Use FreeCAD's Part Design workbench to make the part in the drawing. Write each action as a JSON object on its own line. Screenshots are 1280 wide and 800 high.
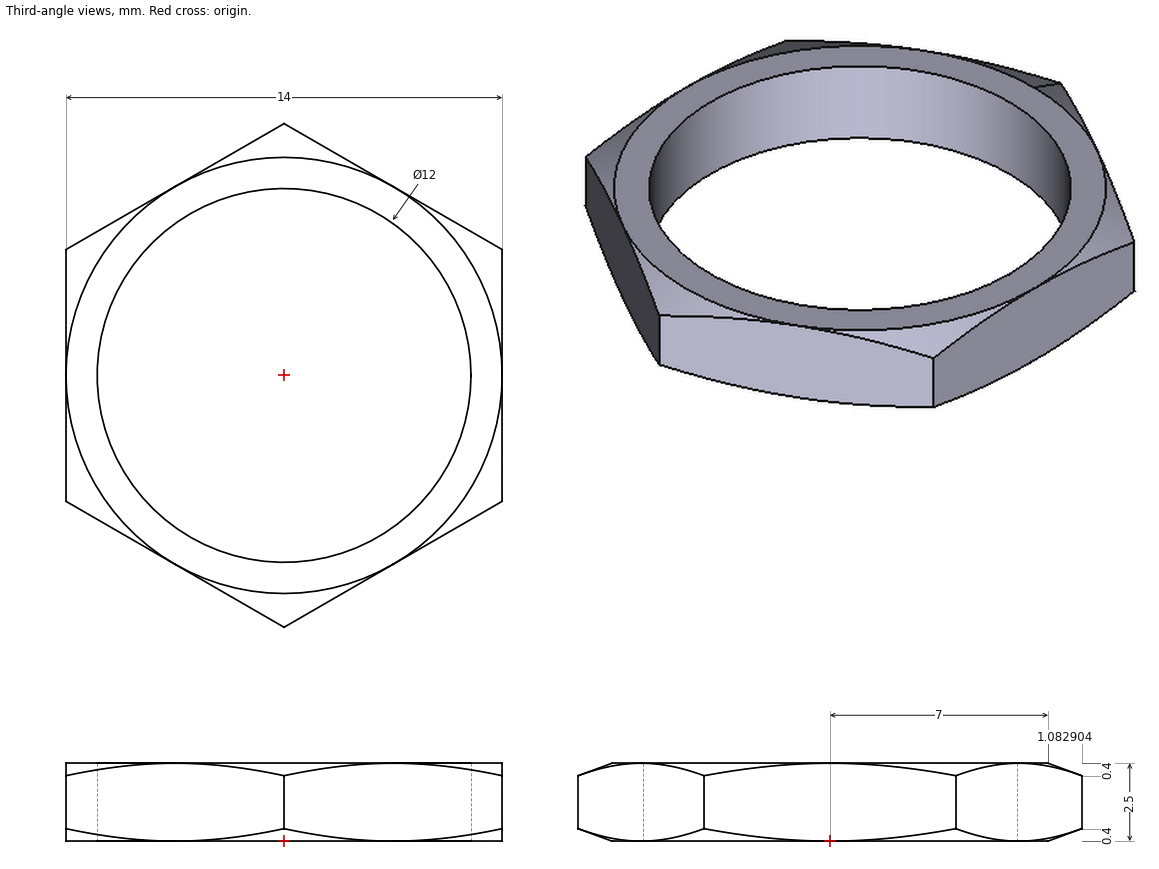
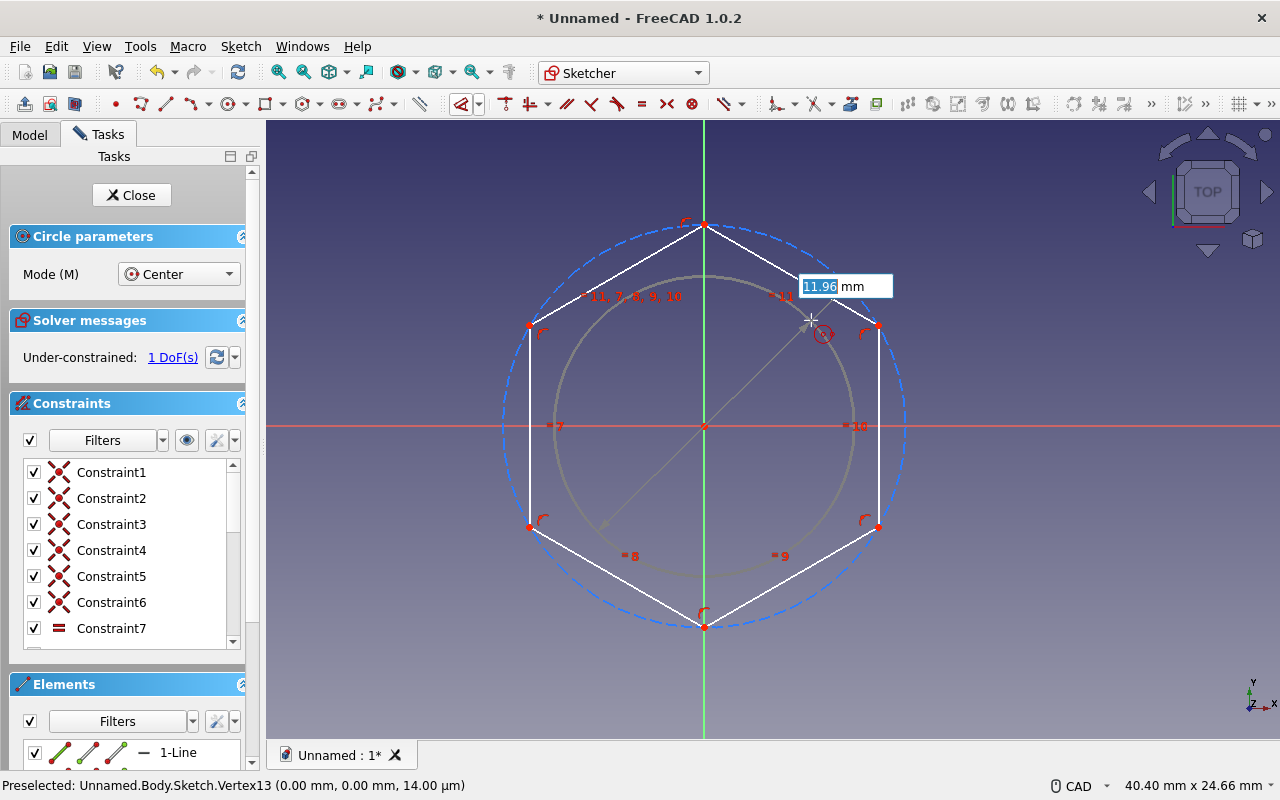
{"action": "type", "text": "12"}
{"action": "key", "text": "Return"}
{"action": "key", "text": "Escape"}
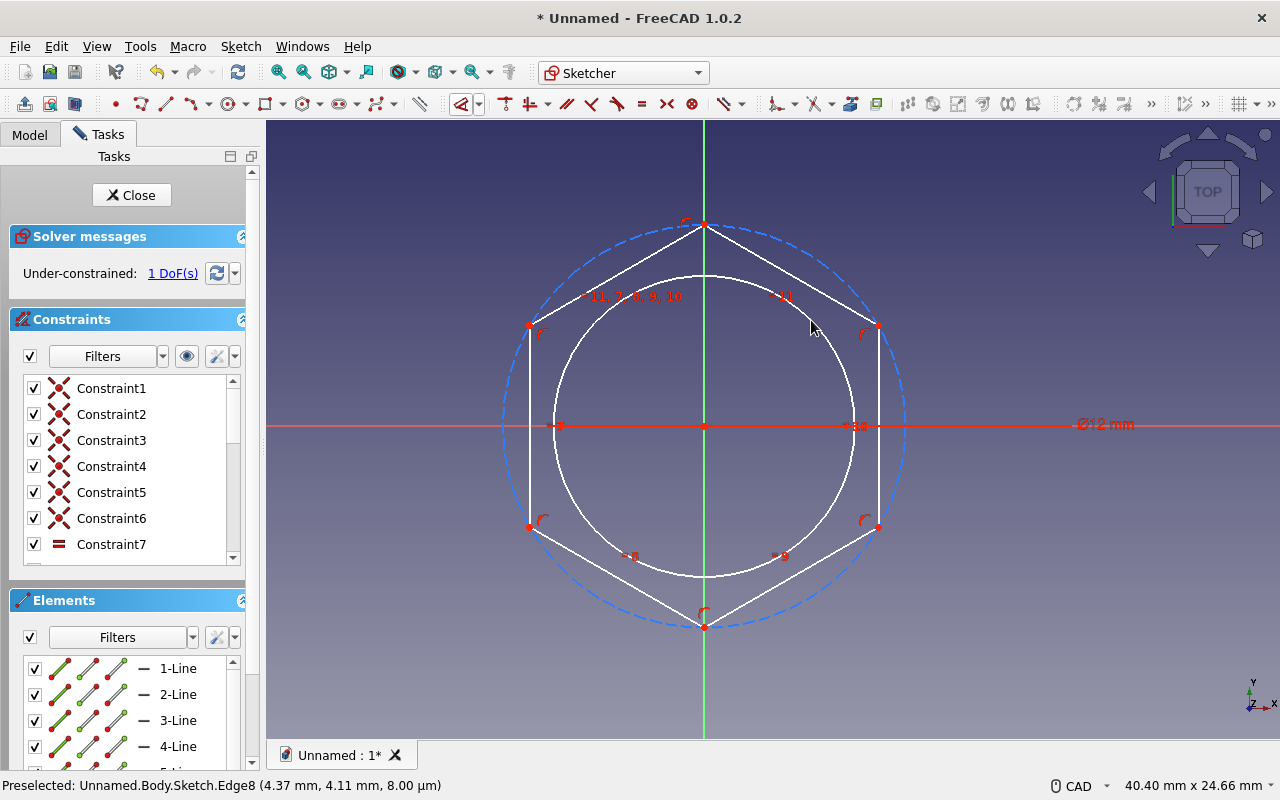
{"action": "left_click", "coordinate": [460, 104]}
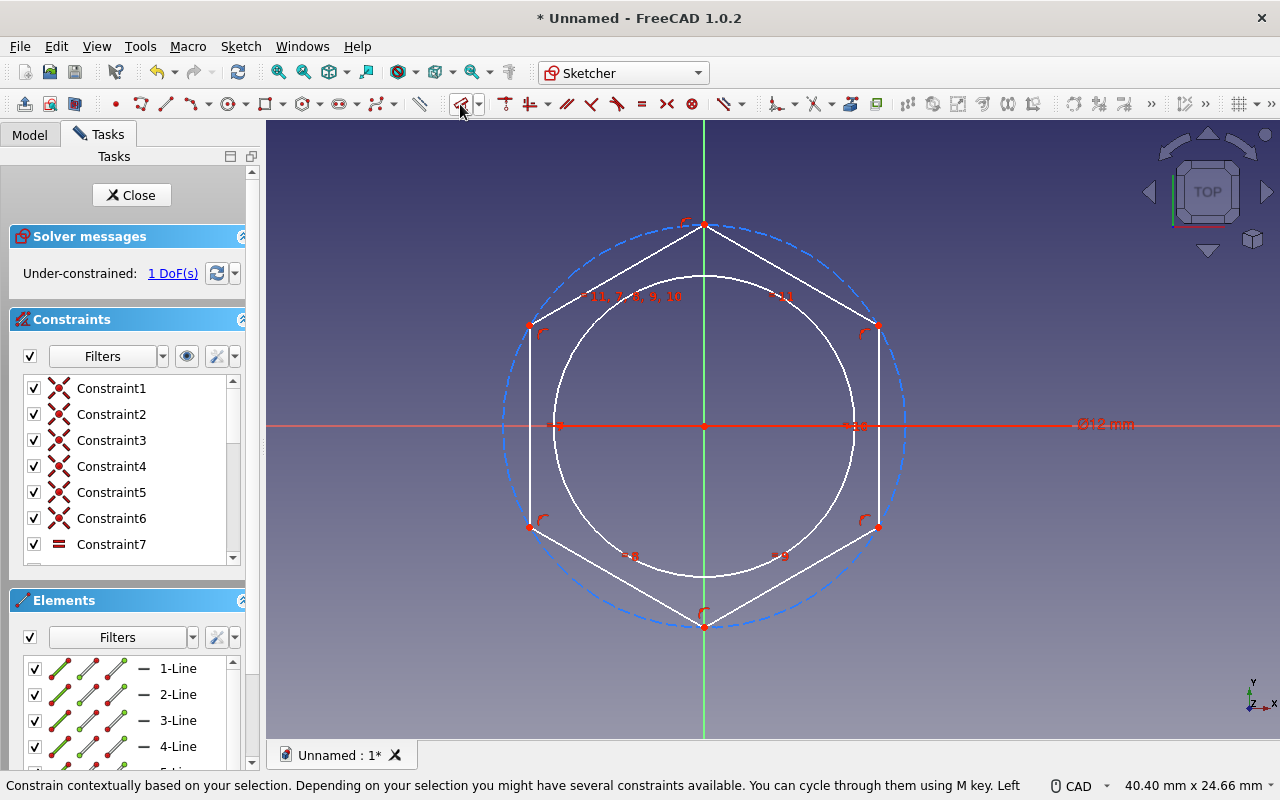
{"action": "left_click", "coordinate": [530, 326]}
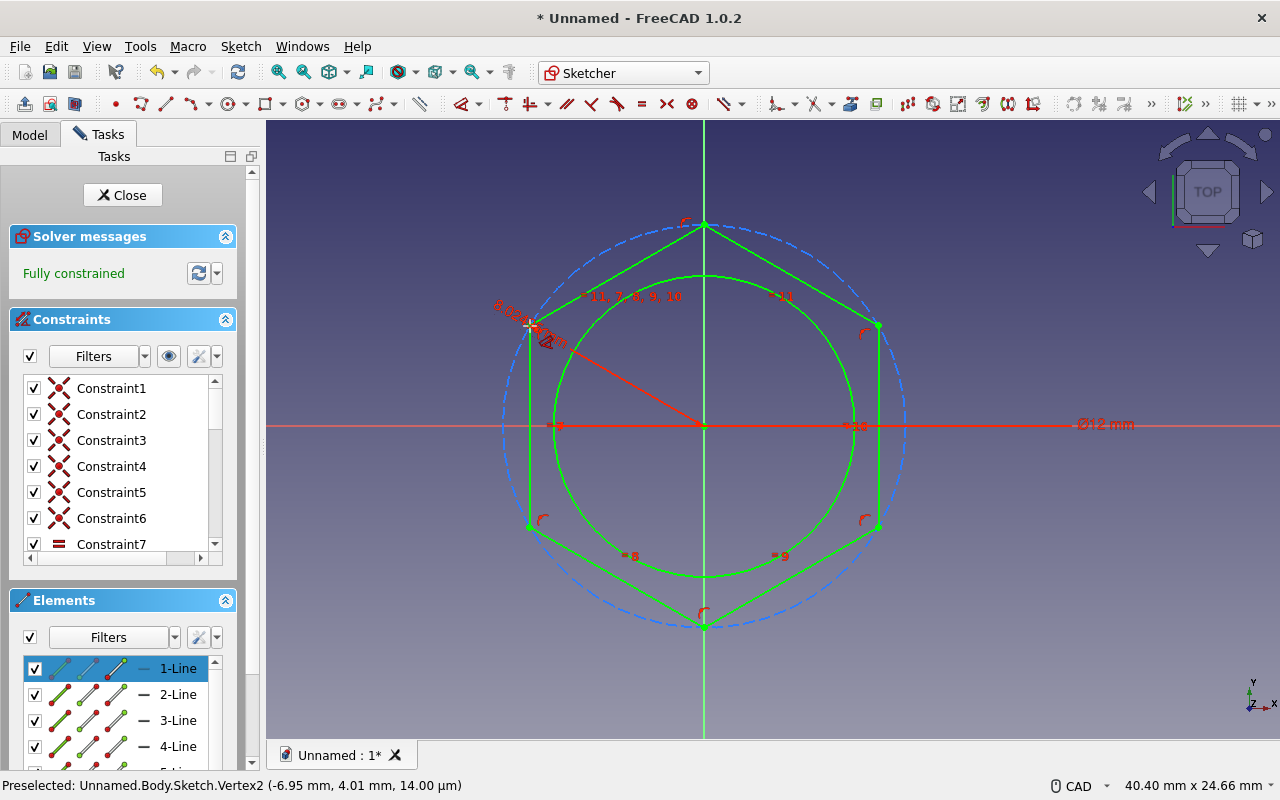
{"action": "left_click", "coordinate": [879, 527]}
{"action": "left_click", "coordinate": [582, 609]}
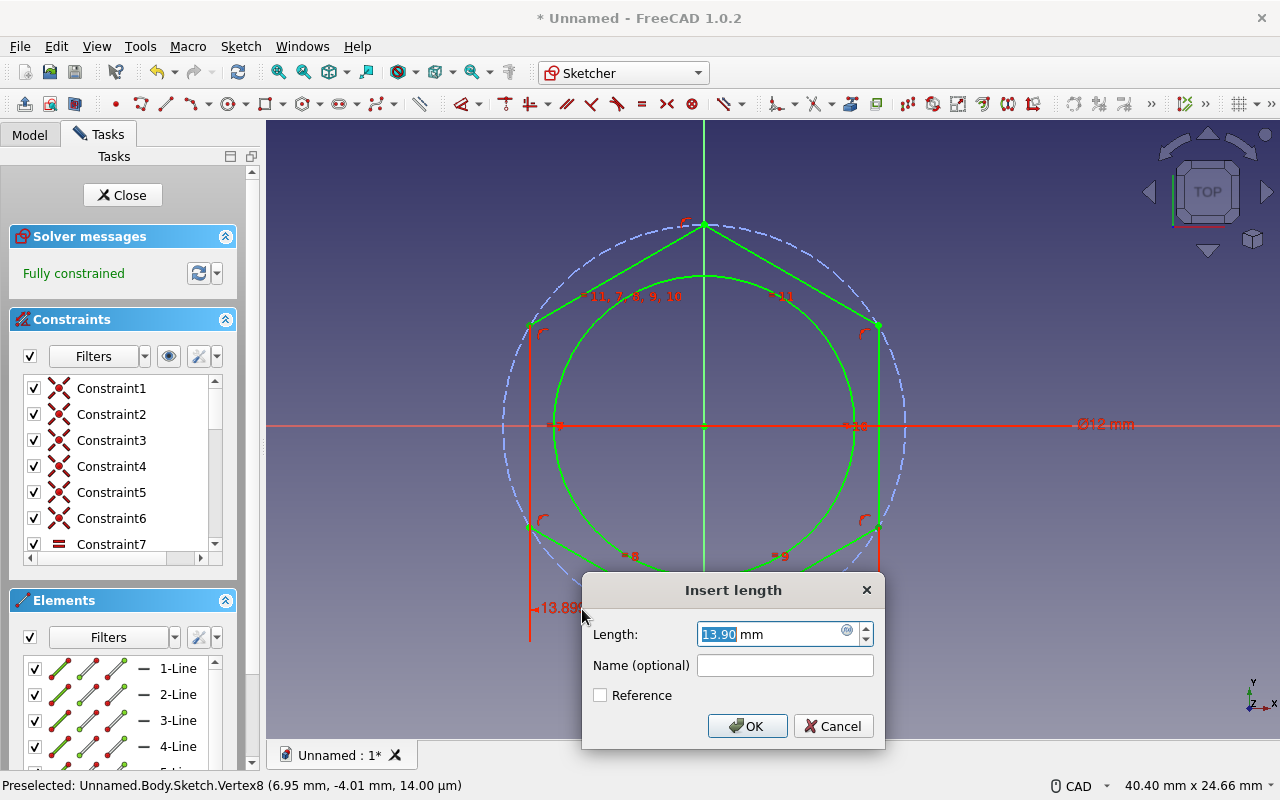
{"action": "type", "text": "14"}
{"action": "key", "text": "Return"}
{"action": "key", "text": "Escape"}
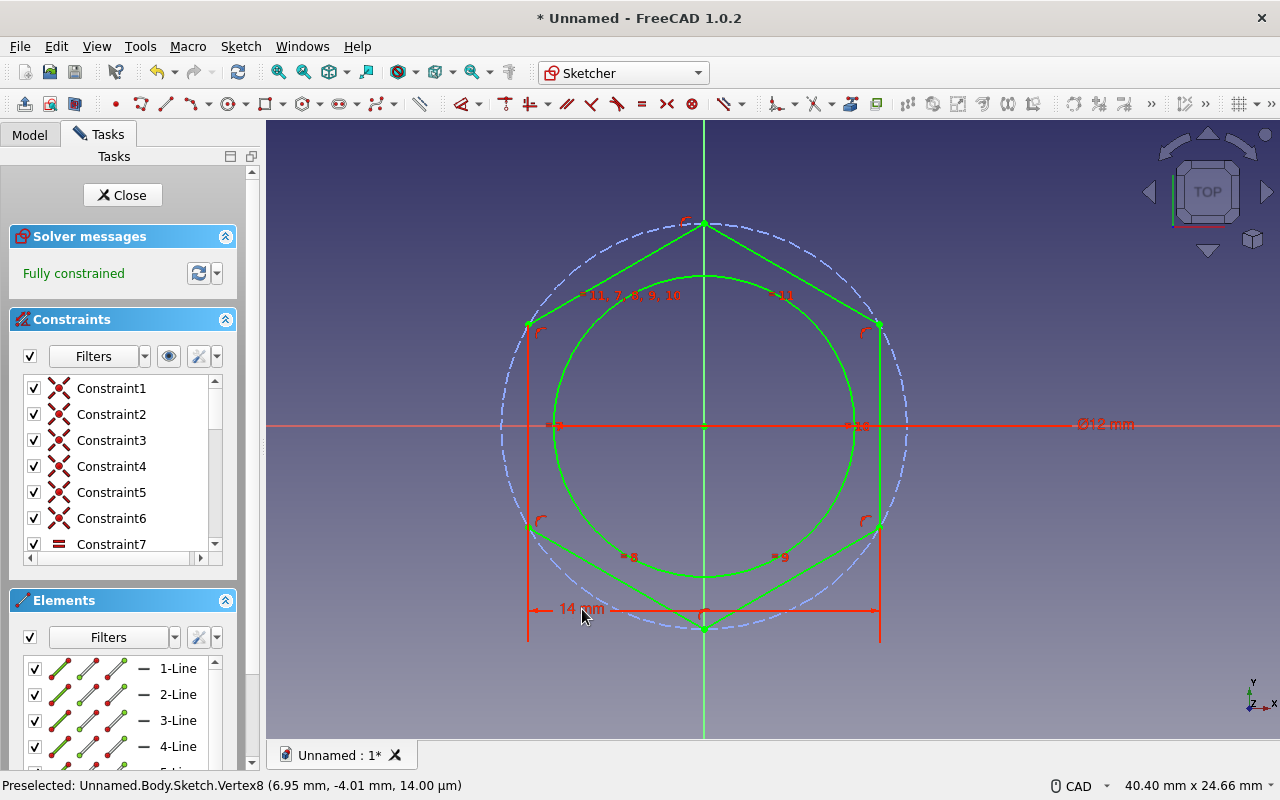
{"action": "left_click", "coordinate": [123, 195]}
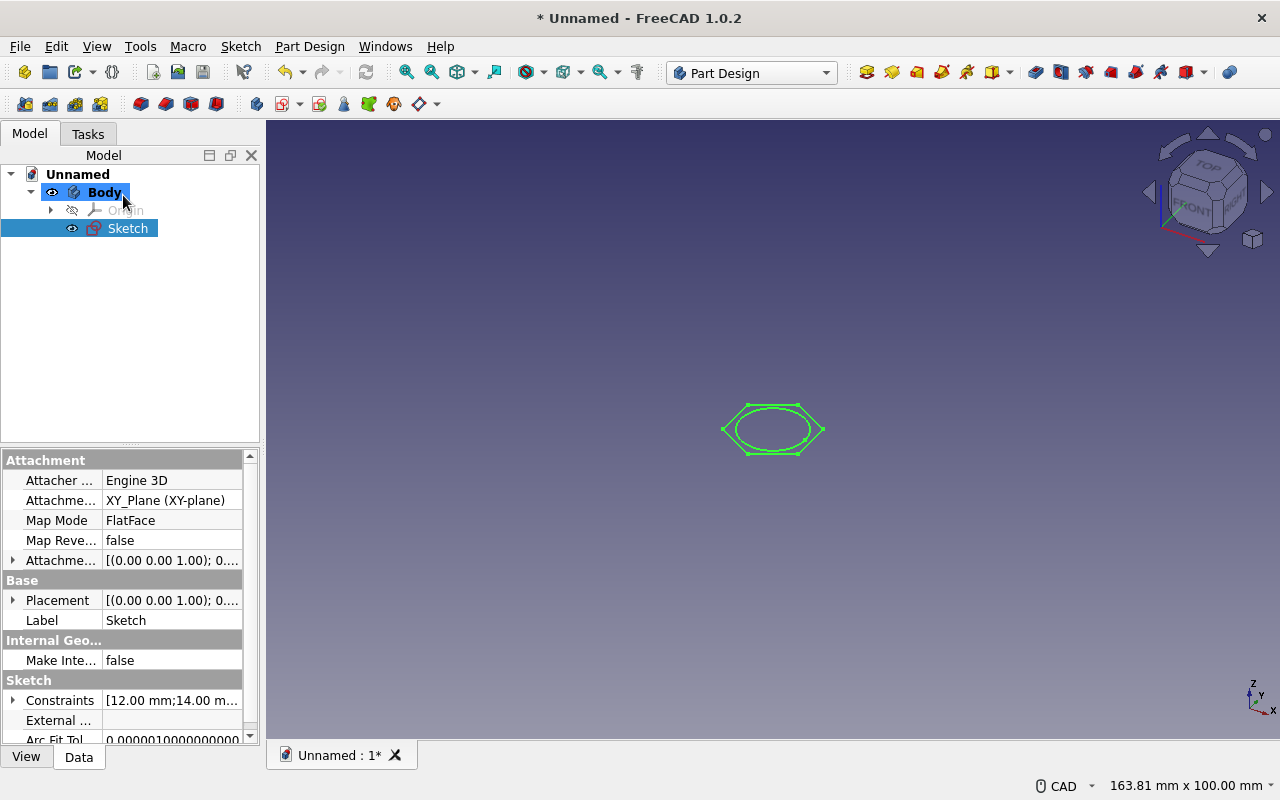
{"action": "left_click", "coordinate": [867, 72]}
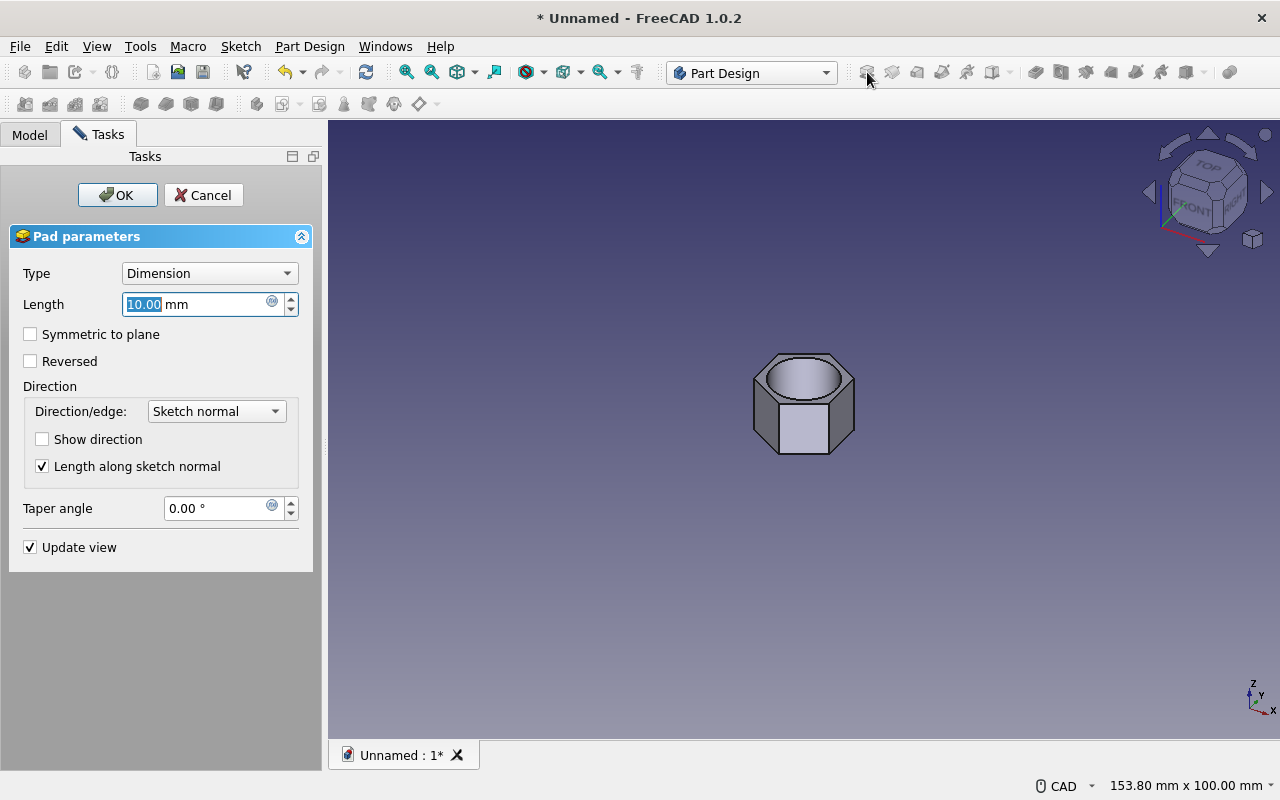
{"action": "type", "text": "2.5"}
{"action": "key", "text": "Tab"}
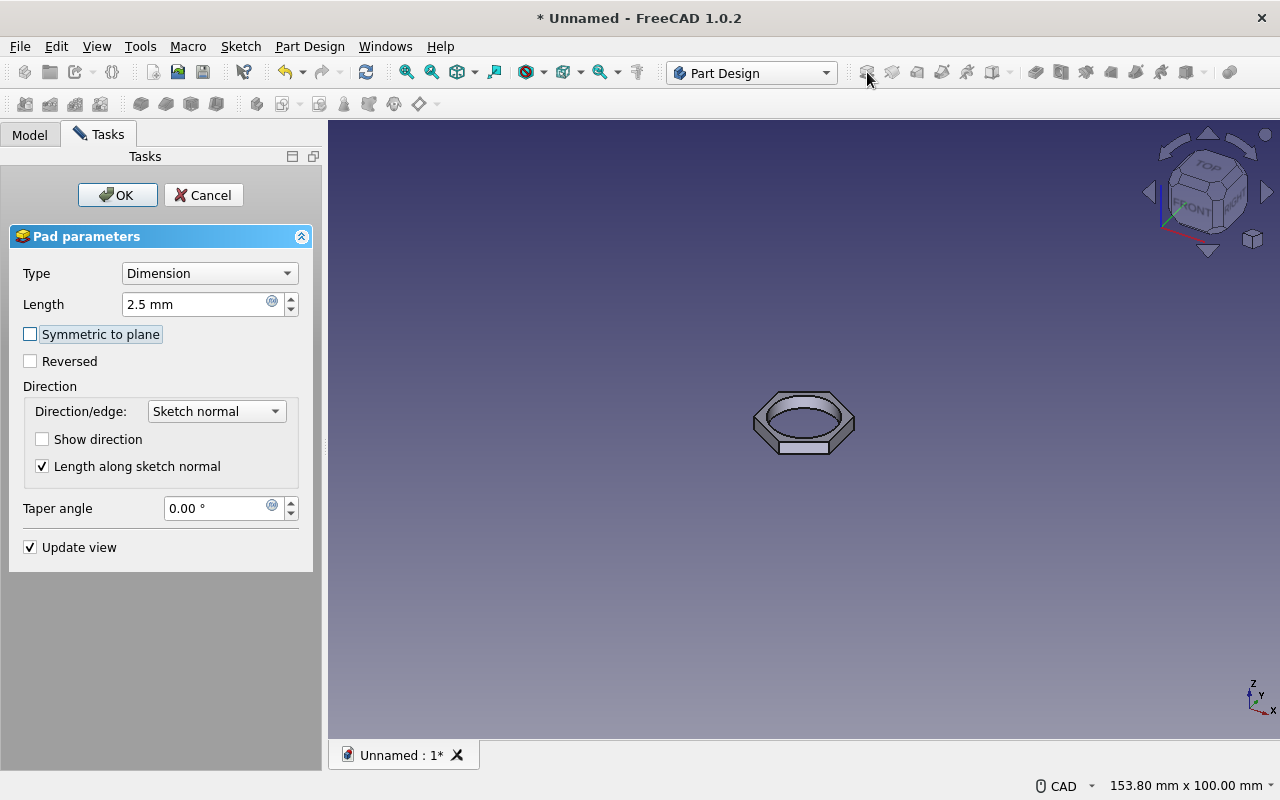
{"action": "left_click", "coordinate": [118, 195]}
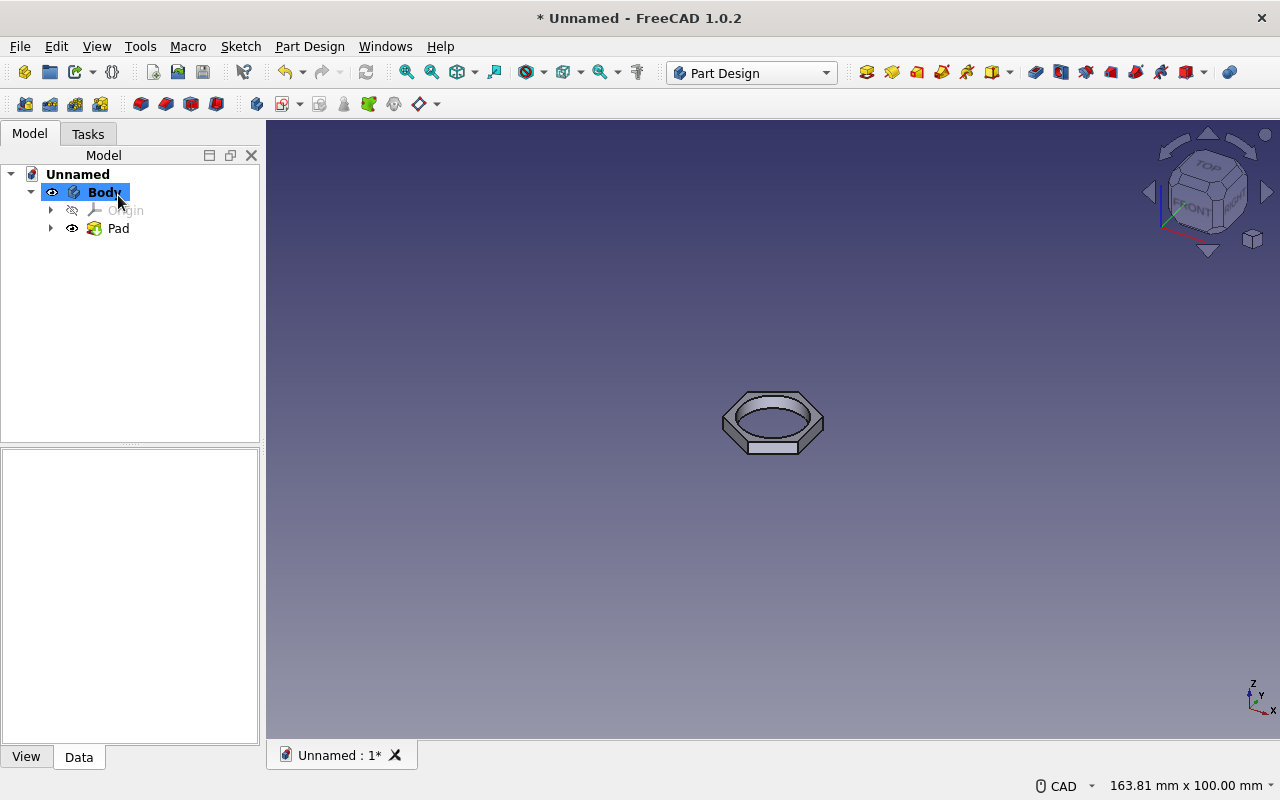
{"action": "key", "text": "v f"}